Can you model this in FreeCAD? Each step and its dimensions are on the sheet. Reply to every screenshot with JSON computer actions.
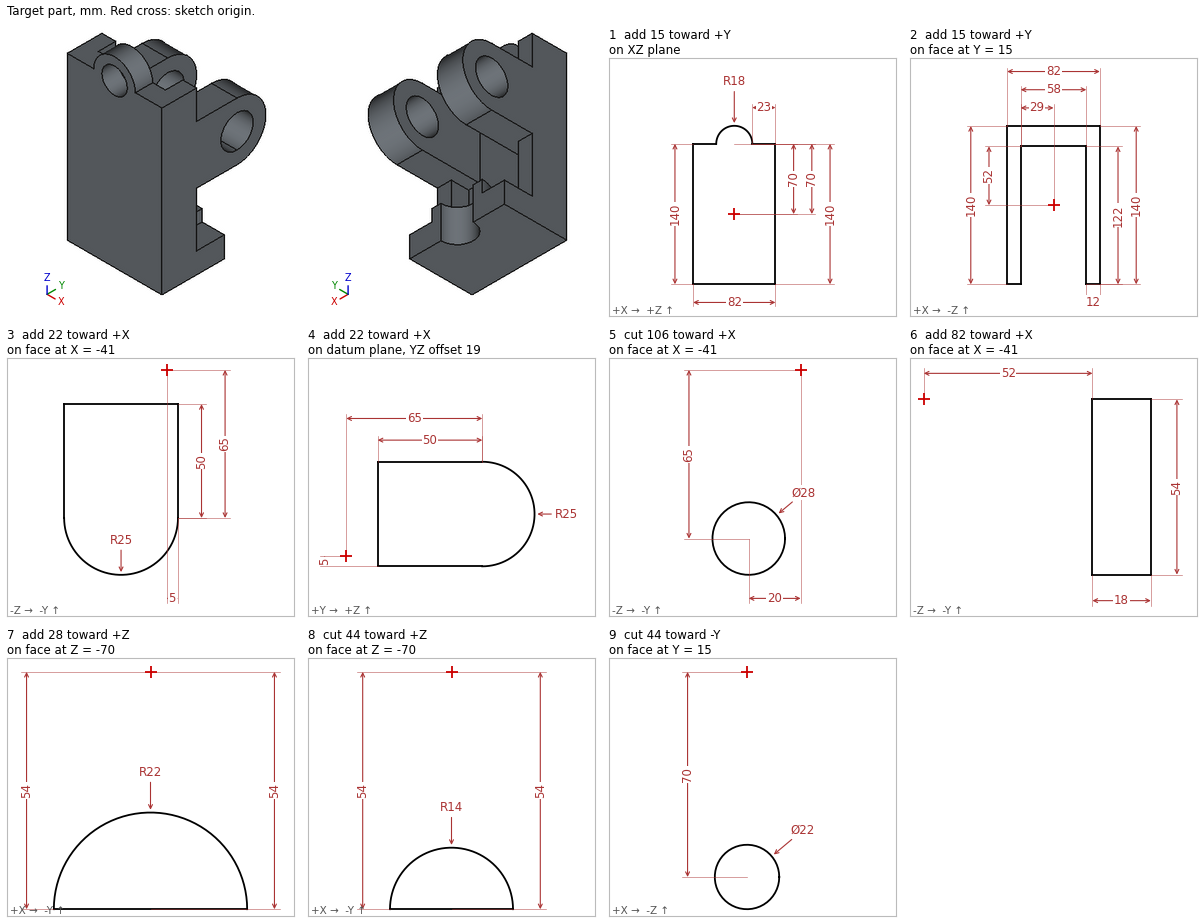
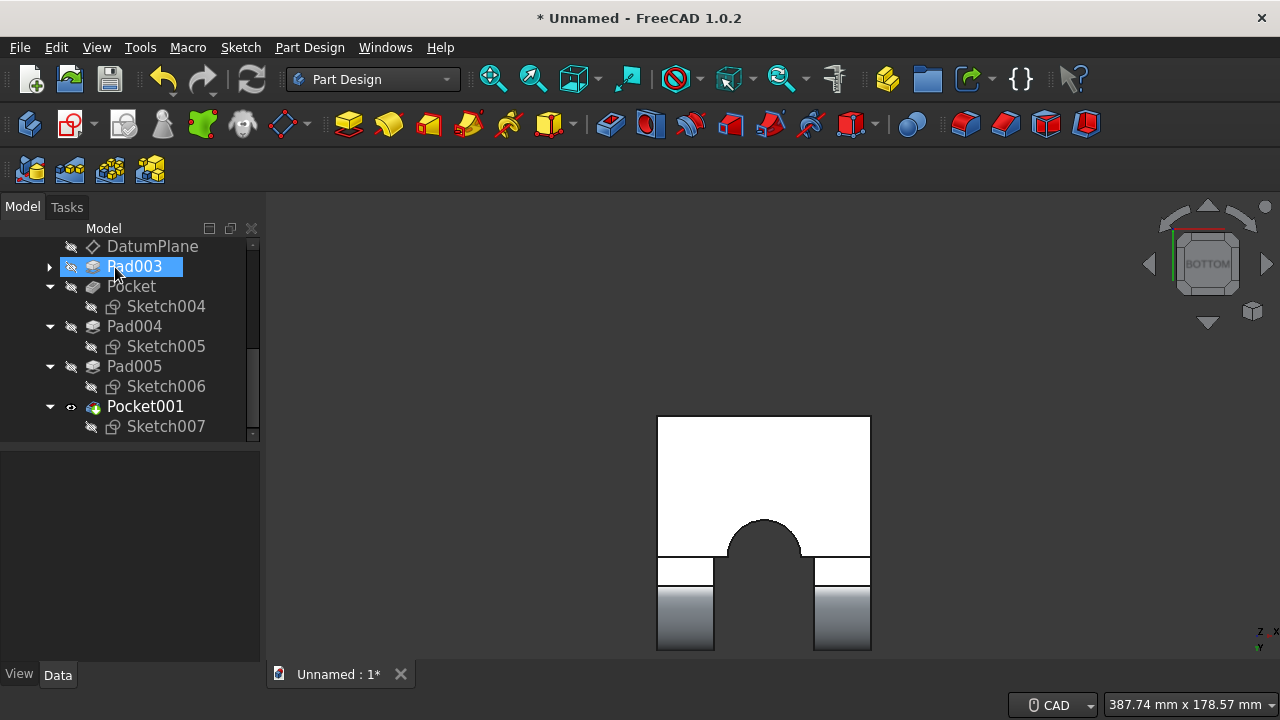
{"action": "key", "text": "4"}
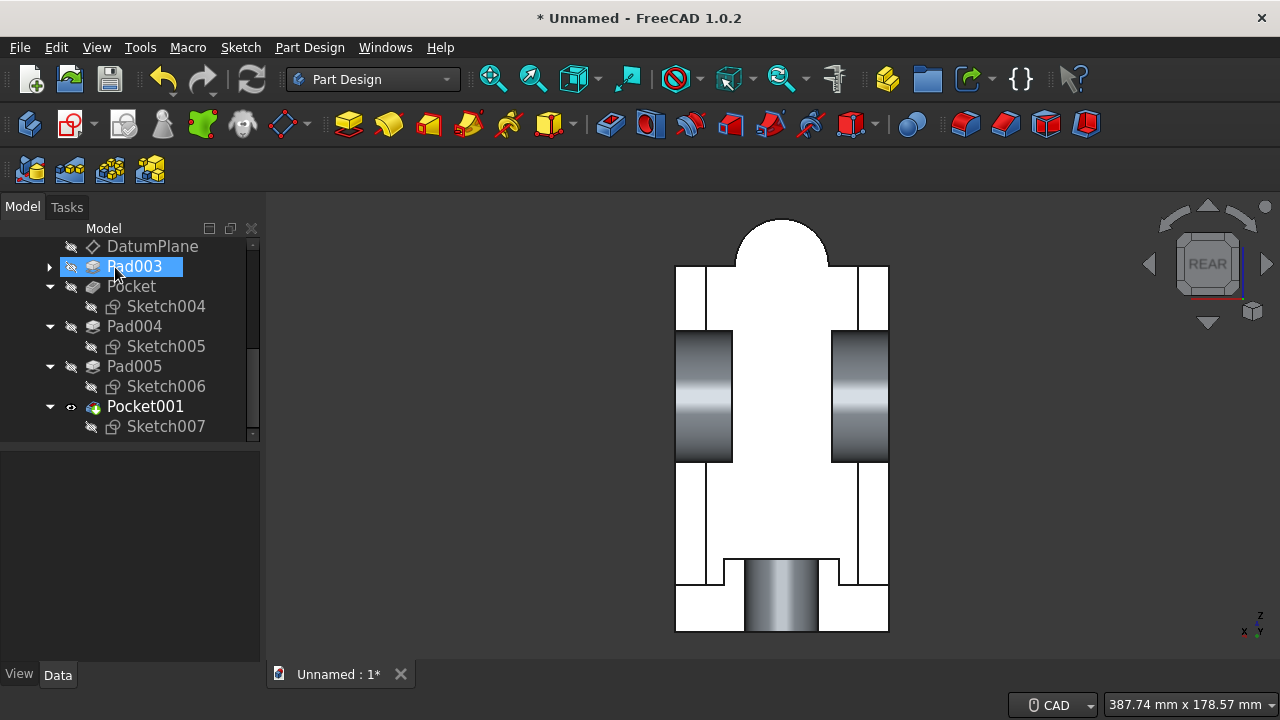
{"action": "left_click", "coordinate": [782, 505]}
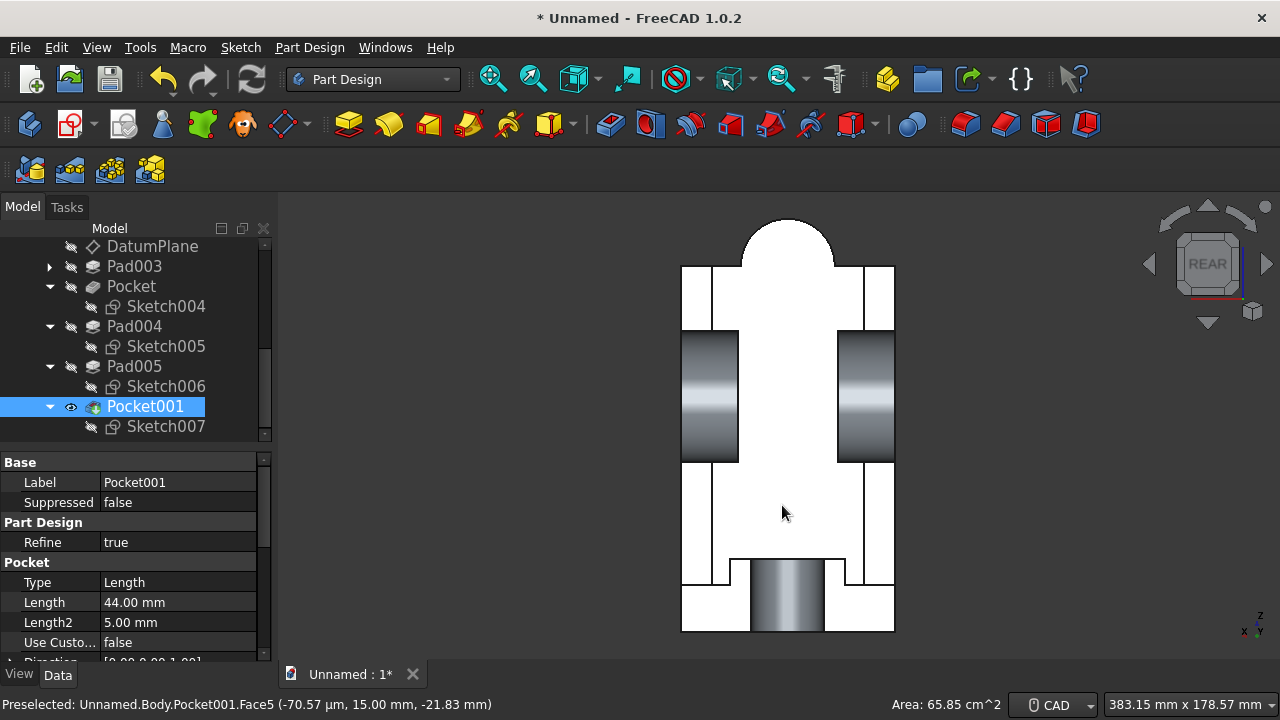
{"action": "left_click", "coordinate": [70, 124]}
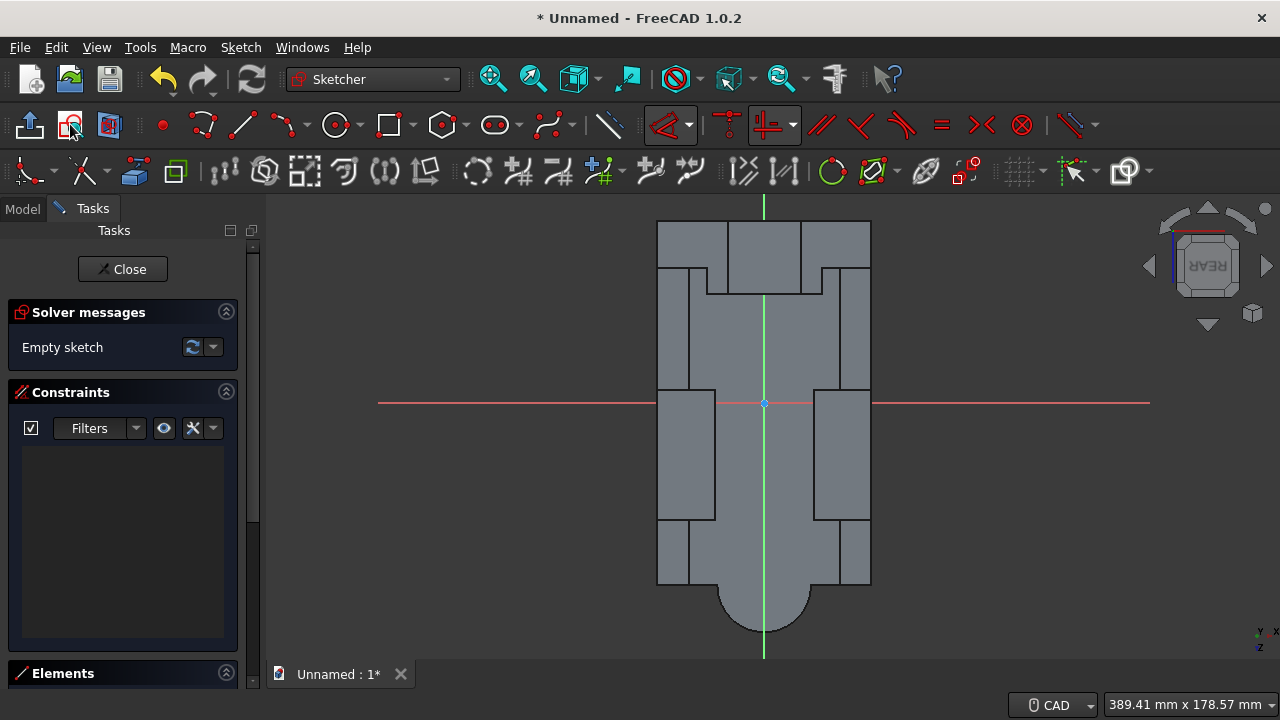
{"action": "scroll", "coordinate": [779, 626], "scroll_direction": "up", "scroll_amount": 8}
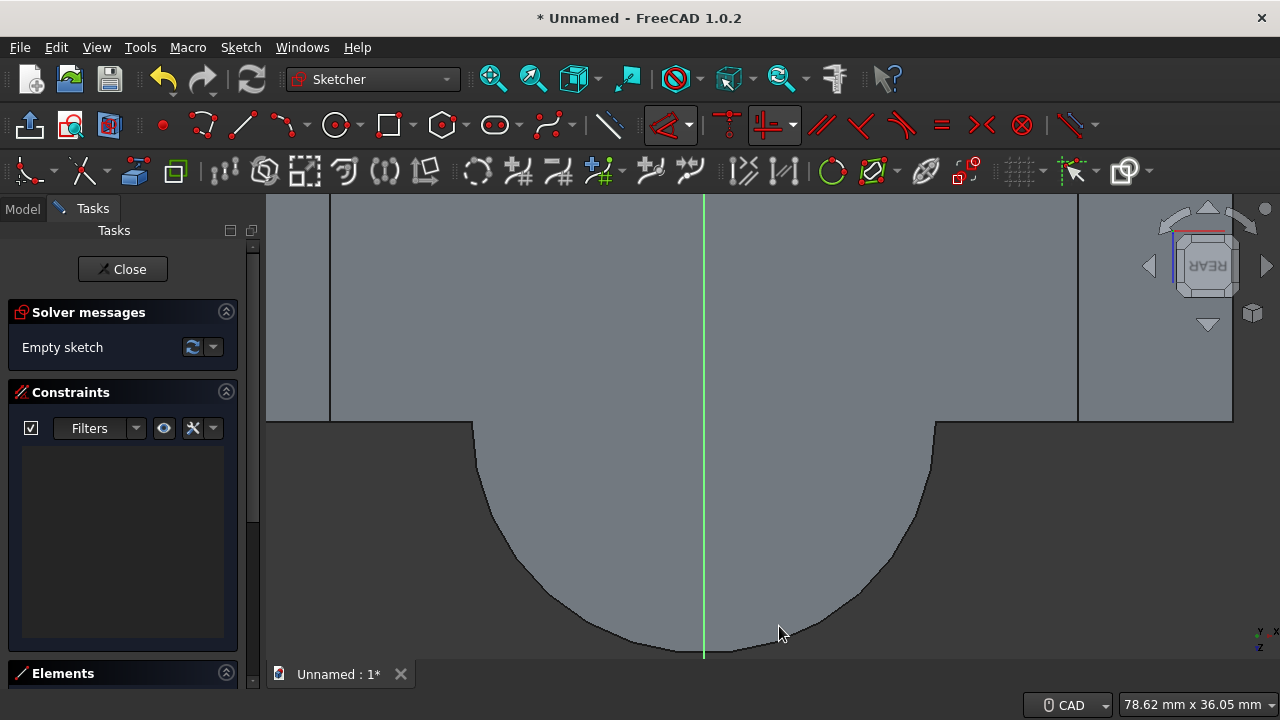
{"action": "key", "text": "g c"}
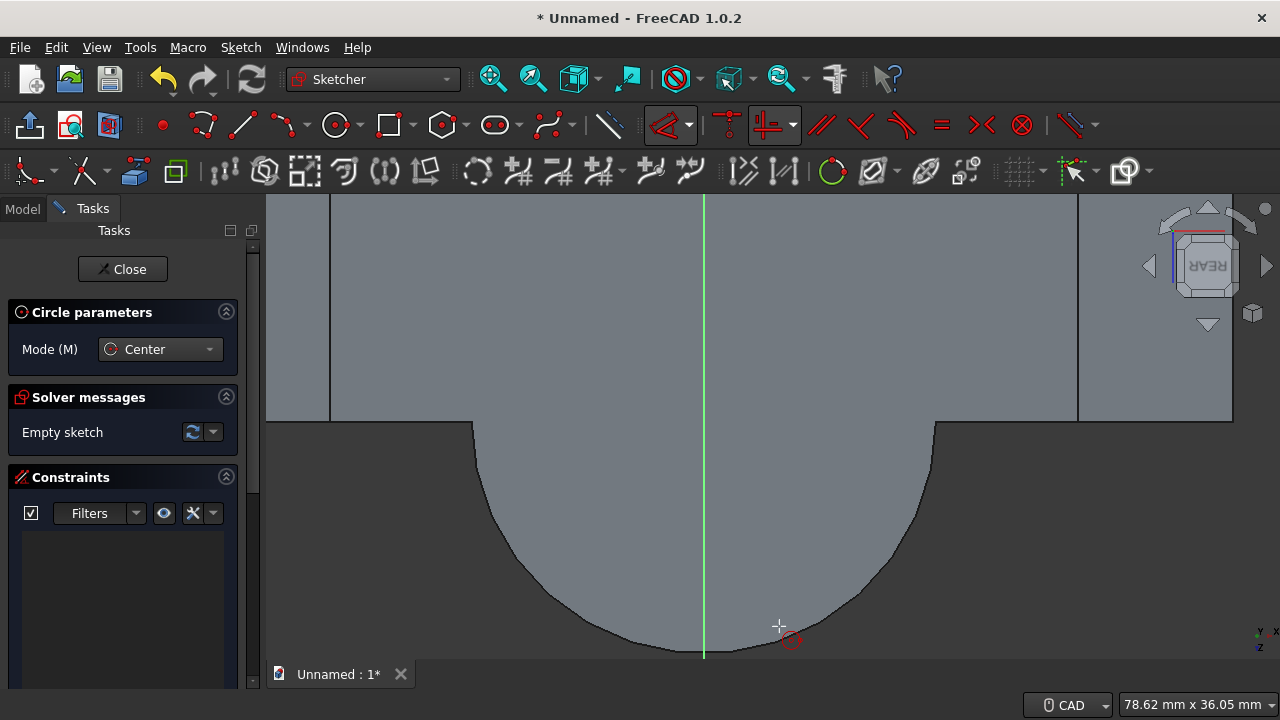
{"action": "left_click", "coordinate": [704, 422]}
{"action": "mouse_move", "coordinate": [804, 321]}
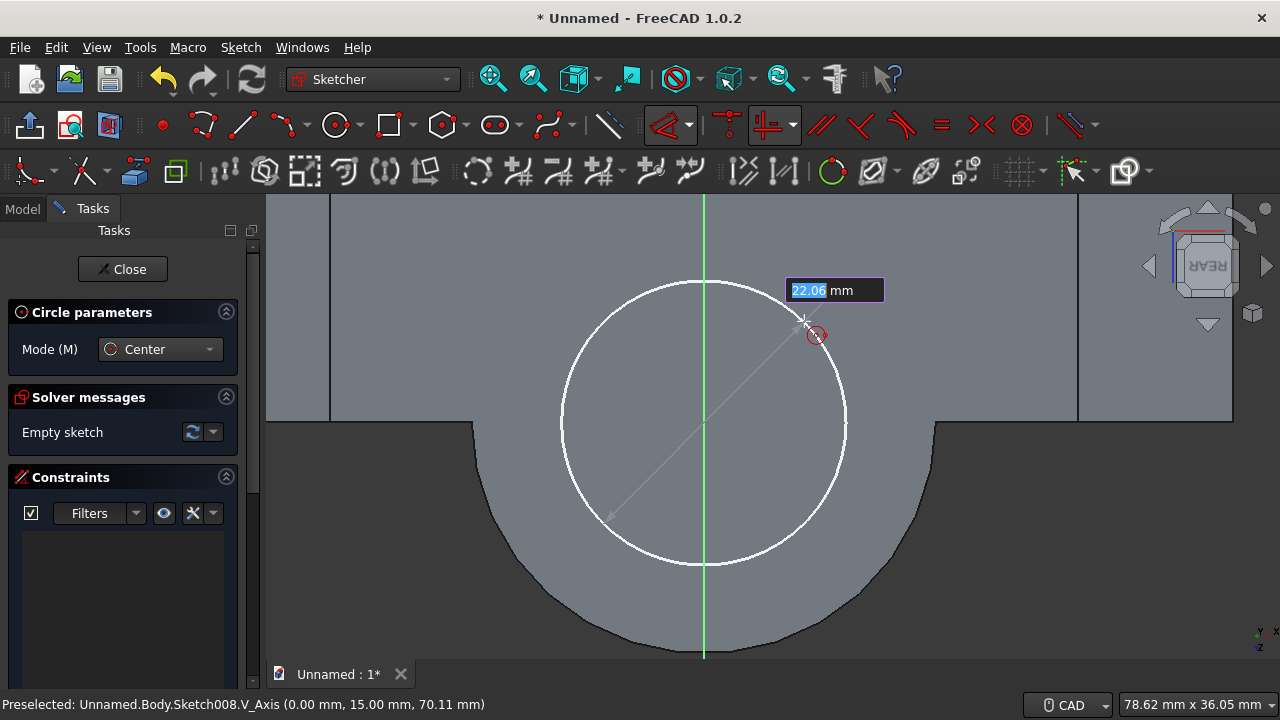
{"action": "type", "text": "22"}
{"action": "key", "text": "Return"}
{"action": "key", "text": "Escape"}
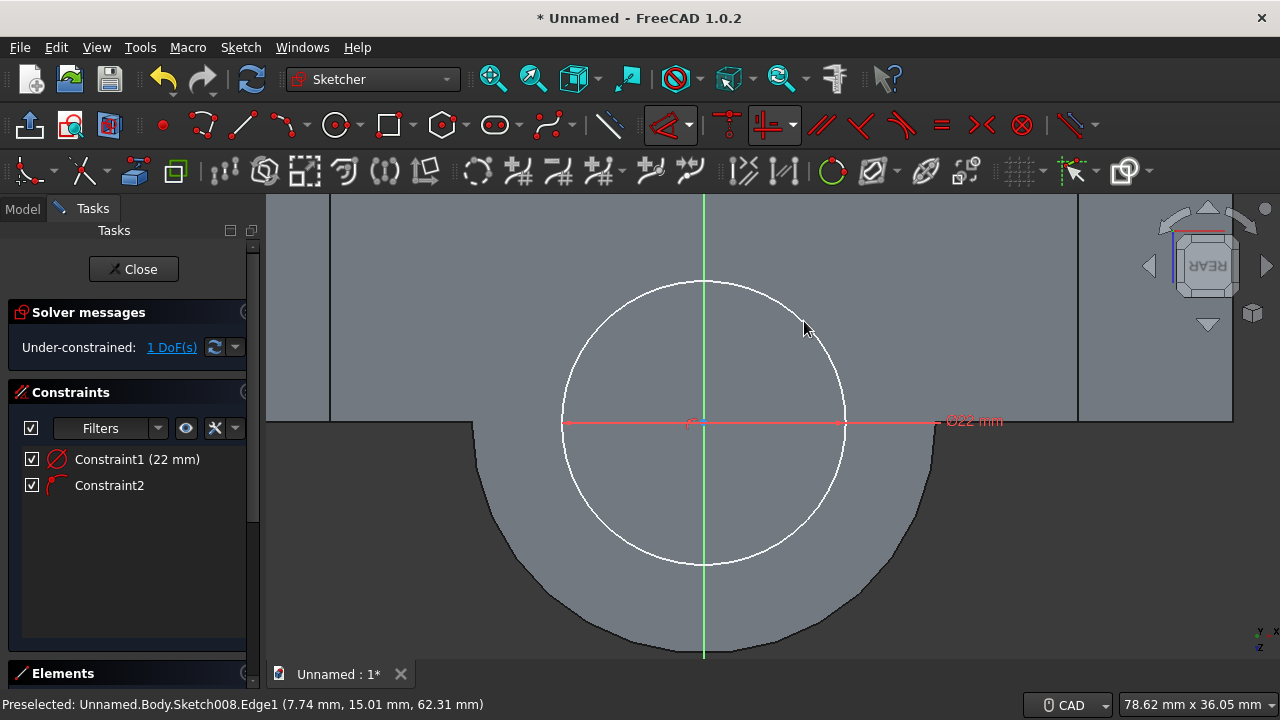
{"action": "left_click", "coordinate": [704, 423]}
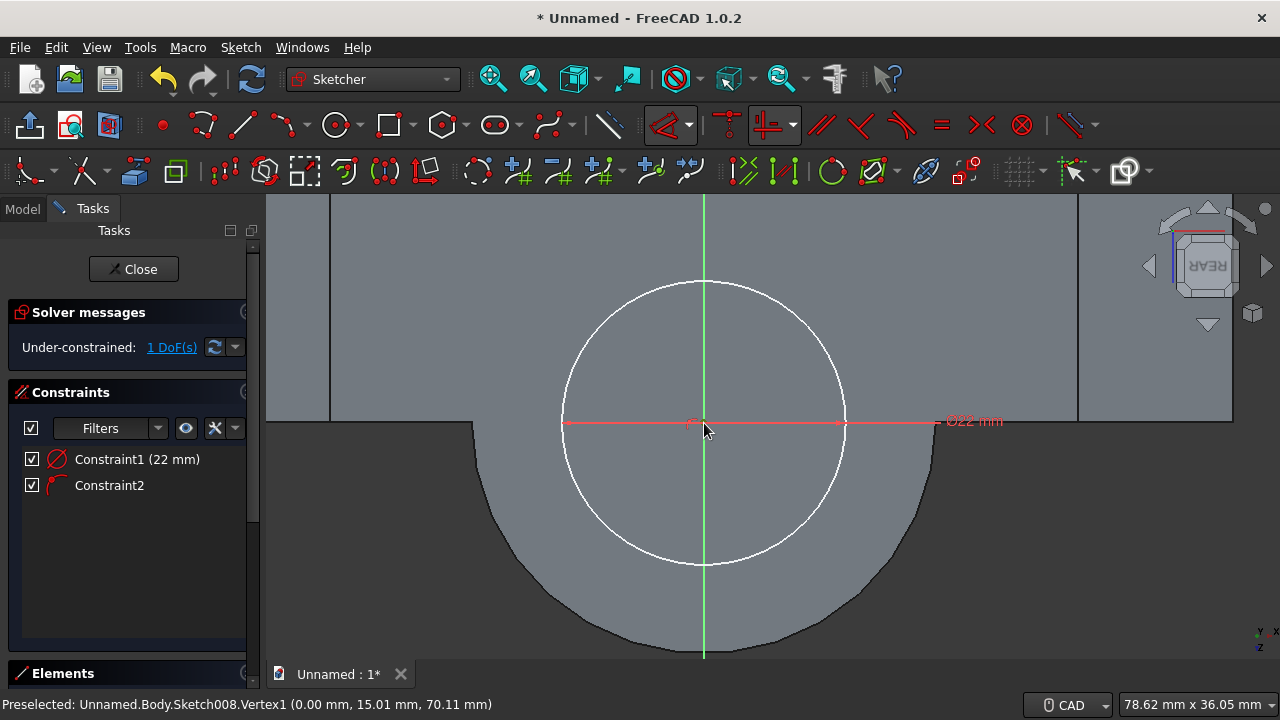
{"action": "left_click", "coordinate": [692, 126]}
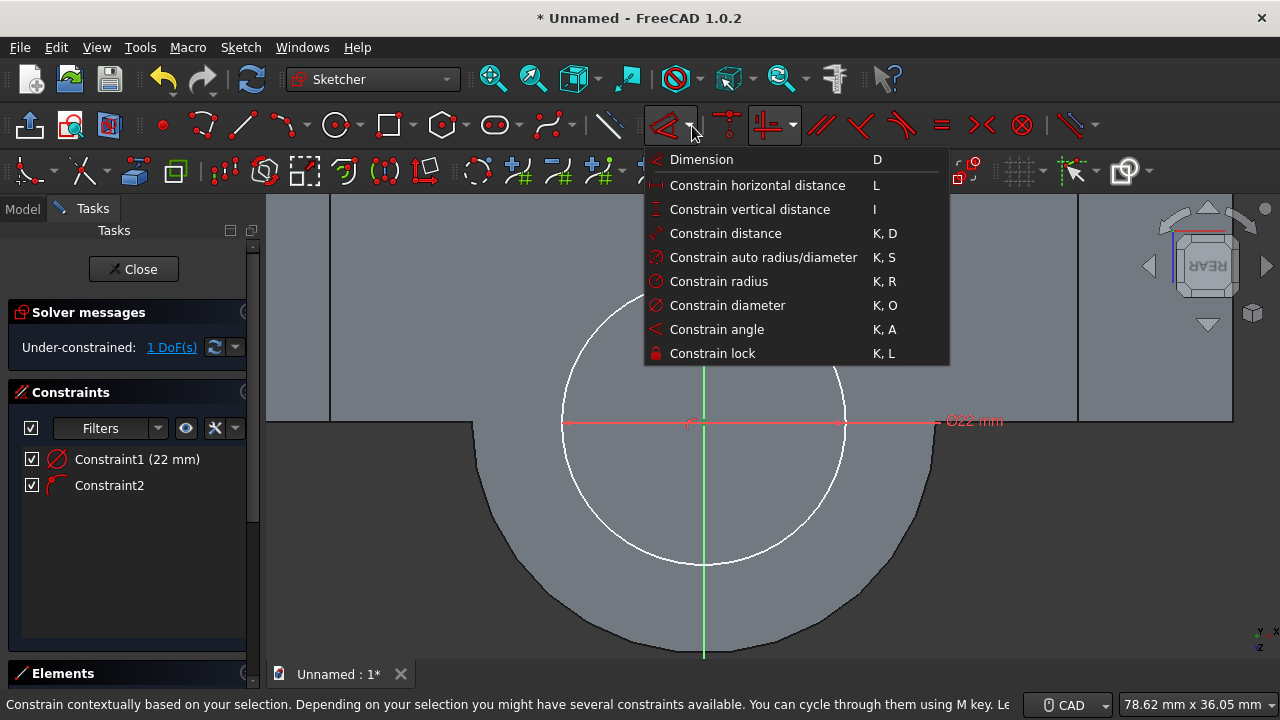
{"action": "left_click", "coordinate": [797, 209]}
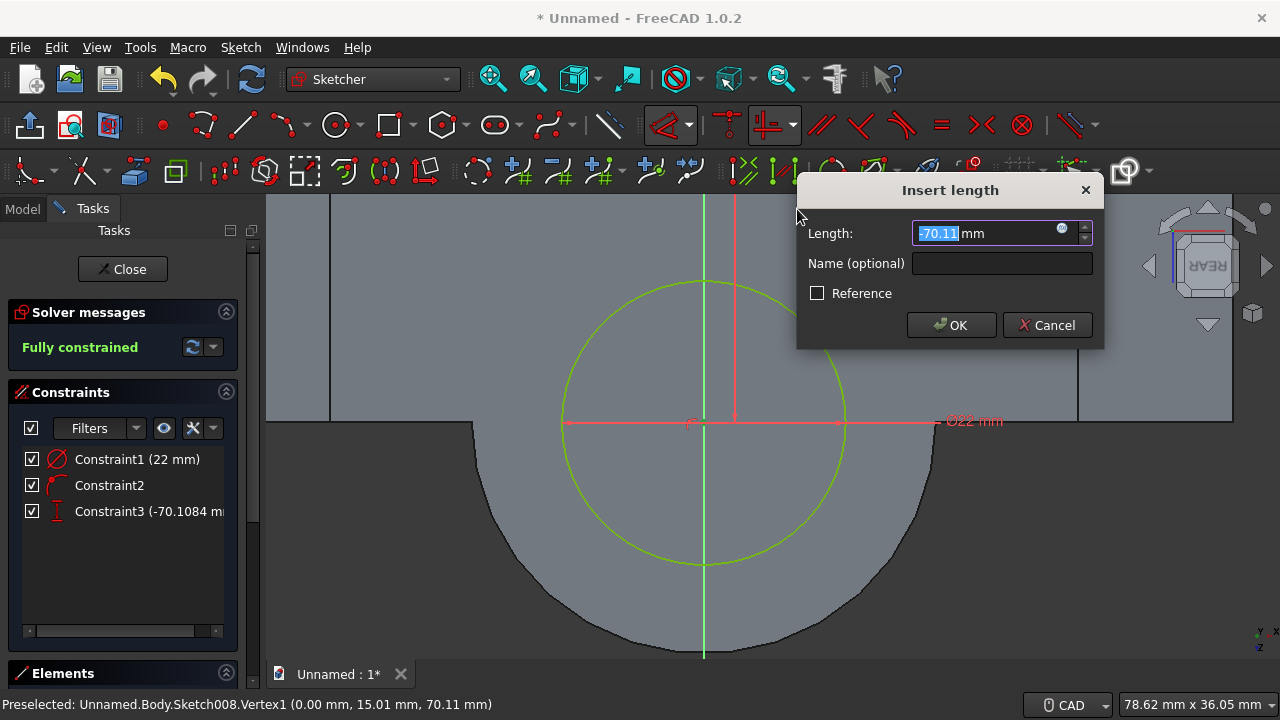
{"action": "type", "text": "-70"}
{"action": "key", "text": "Return"}